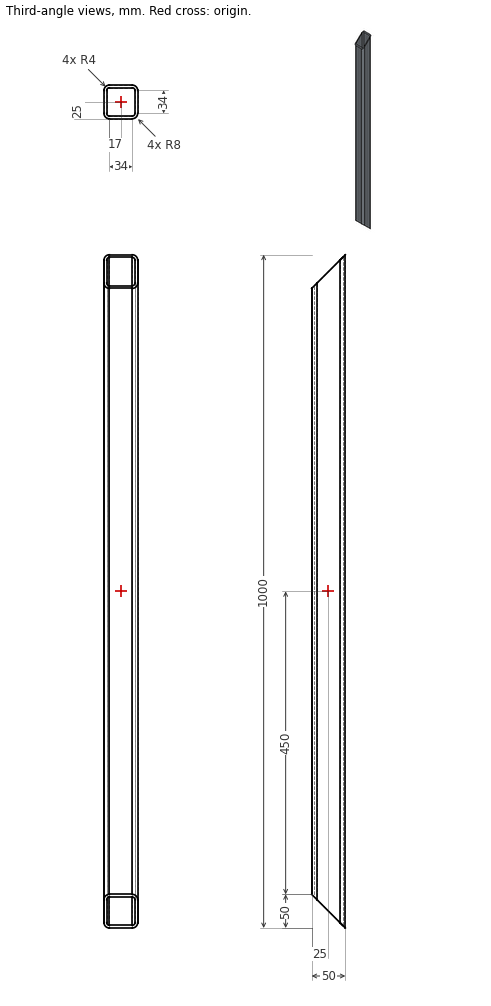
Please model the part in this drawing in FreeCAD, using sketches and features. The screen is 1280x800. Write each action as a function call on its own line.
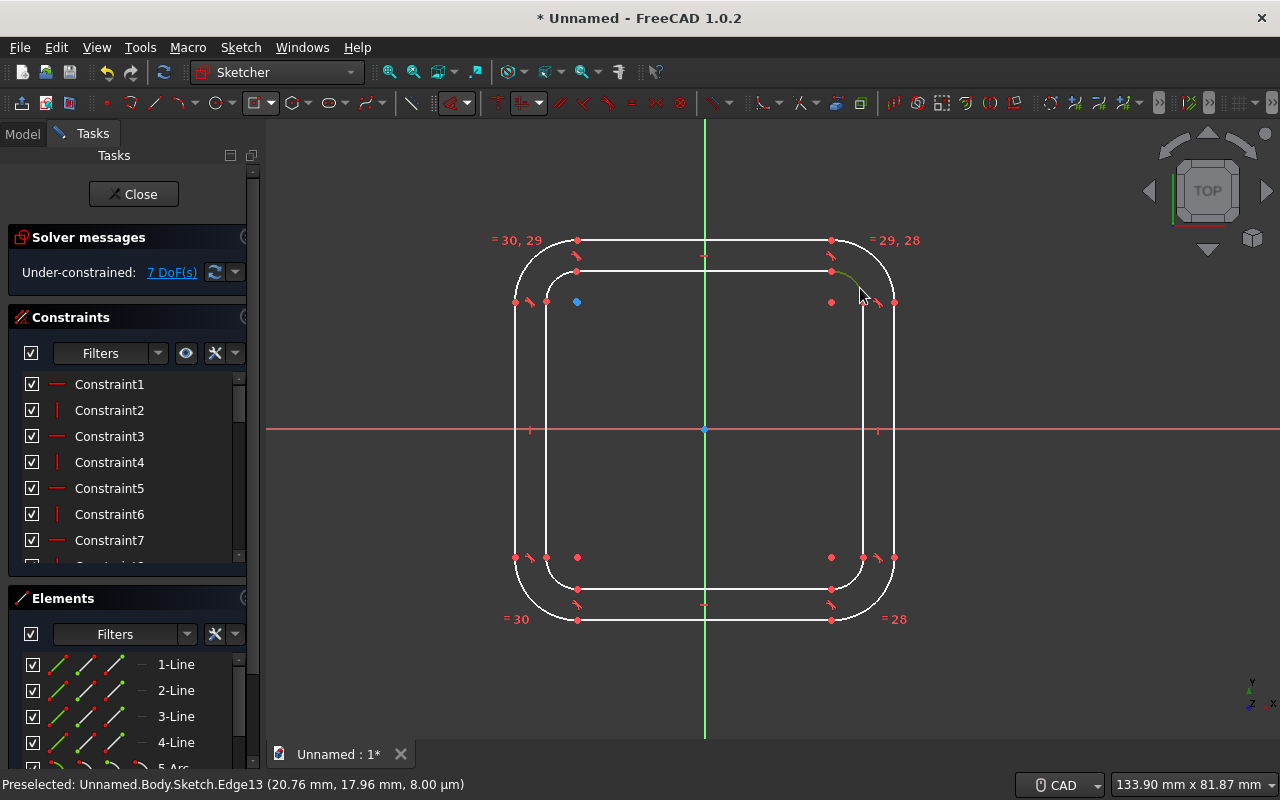
click(563, 275)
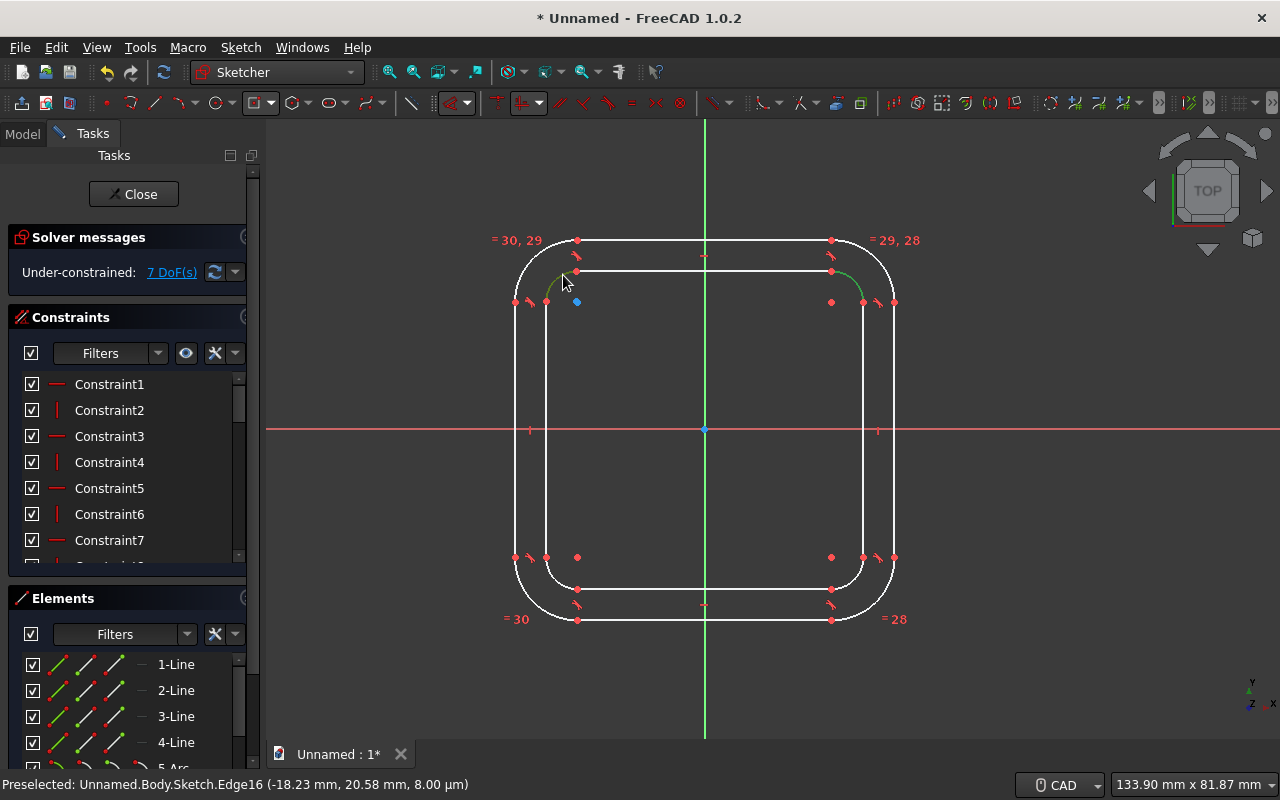
key(e)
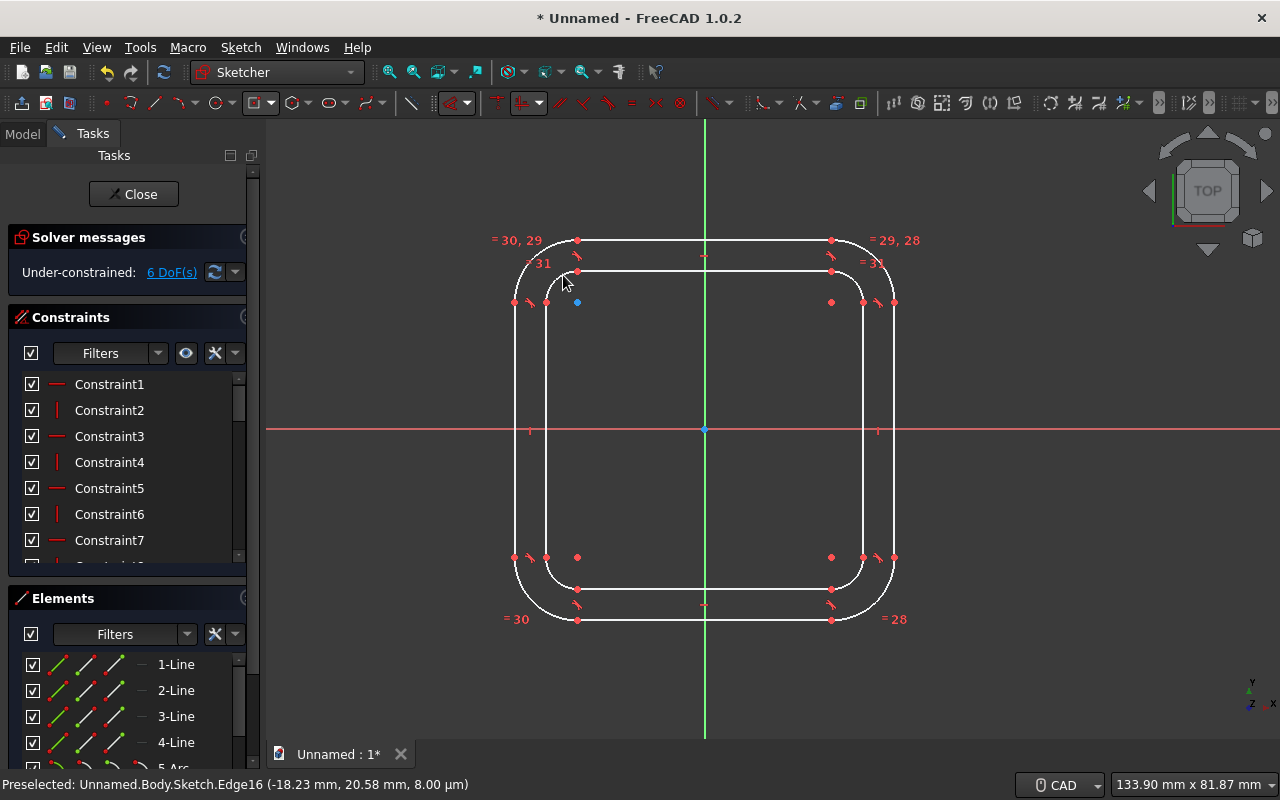
key(d)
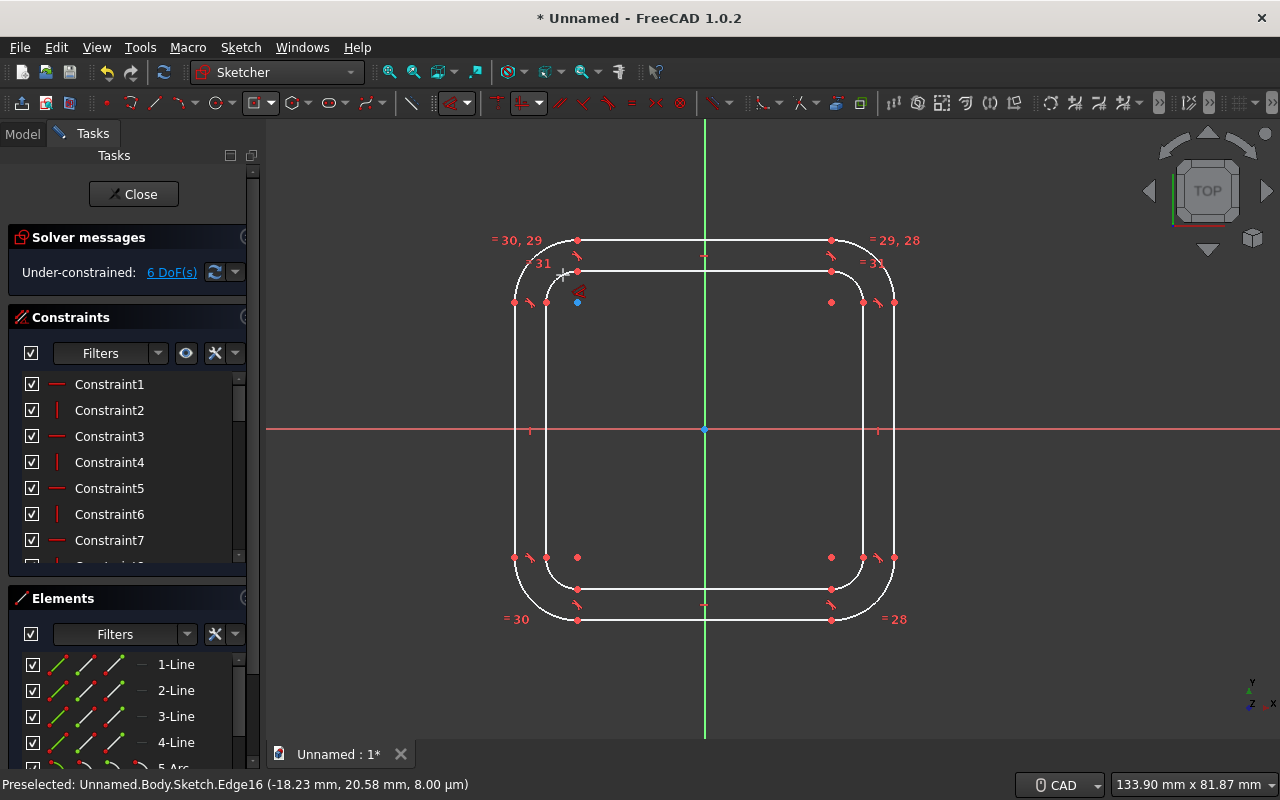
click(860, 614)
click(874, 643)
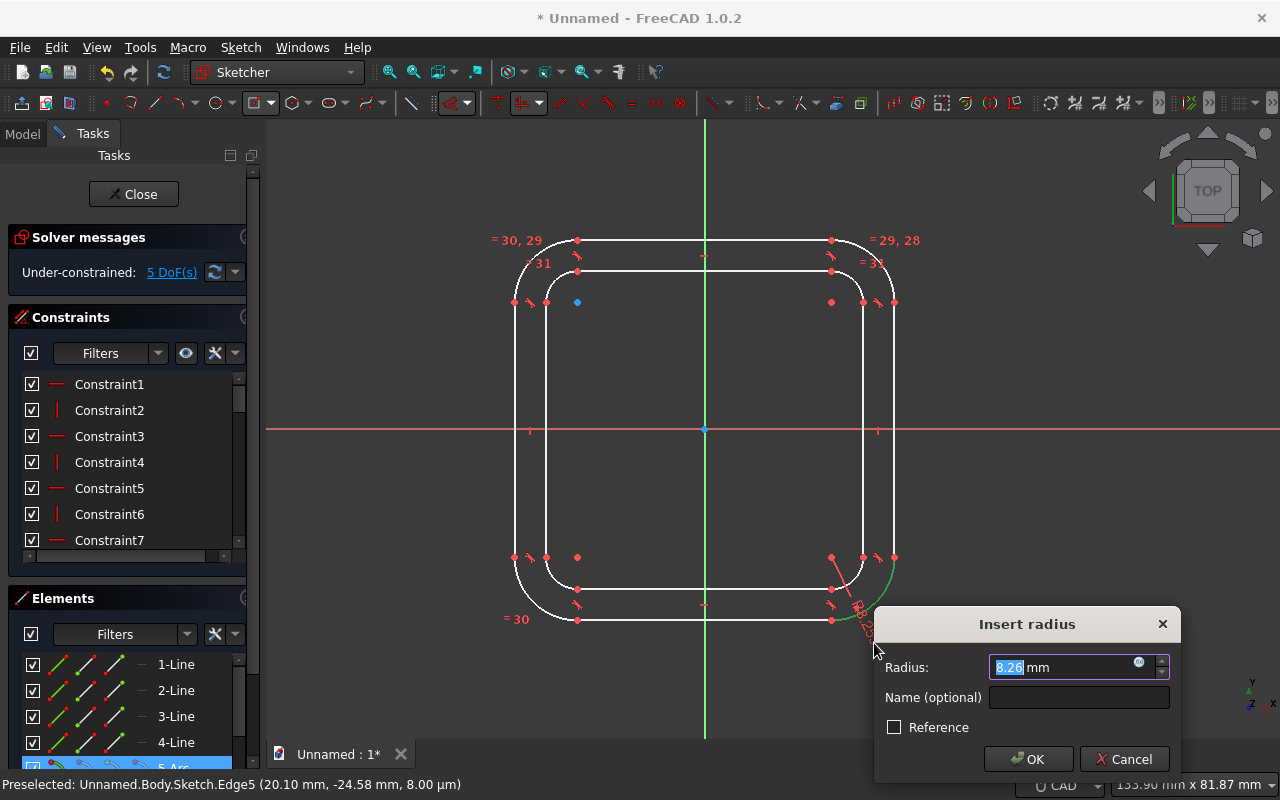
text(8)
key(Return)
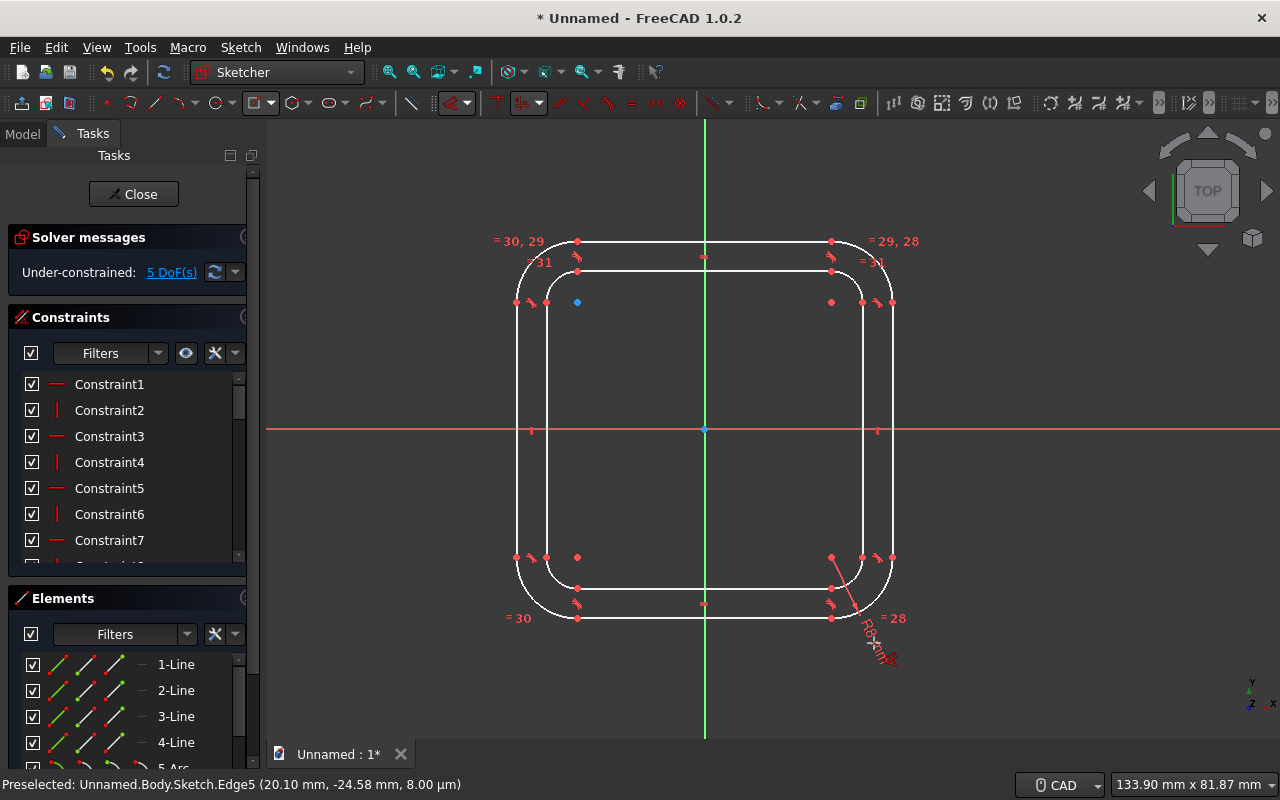
scroll(859, 288, up, 2)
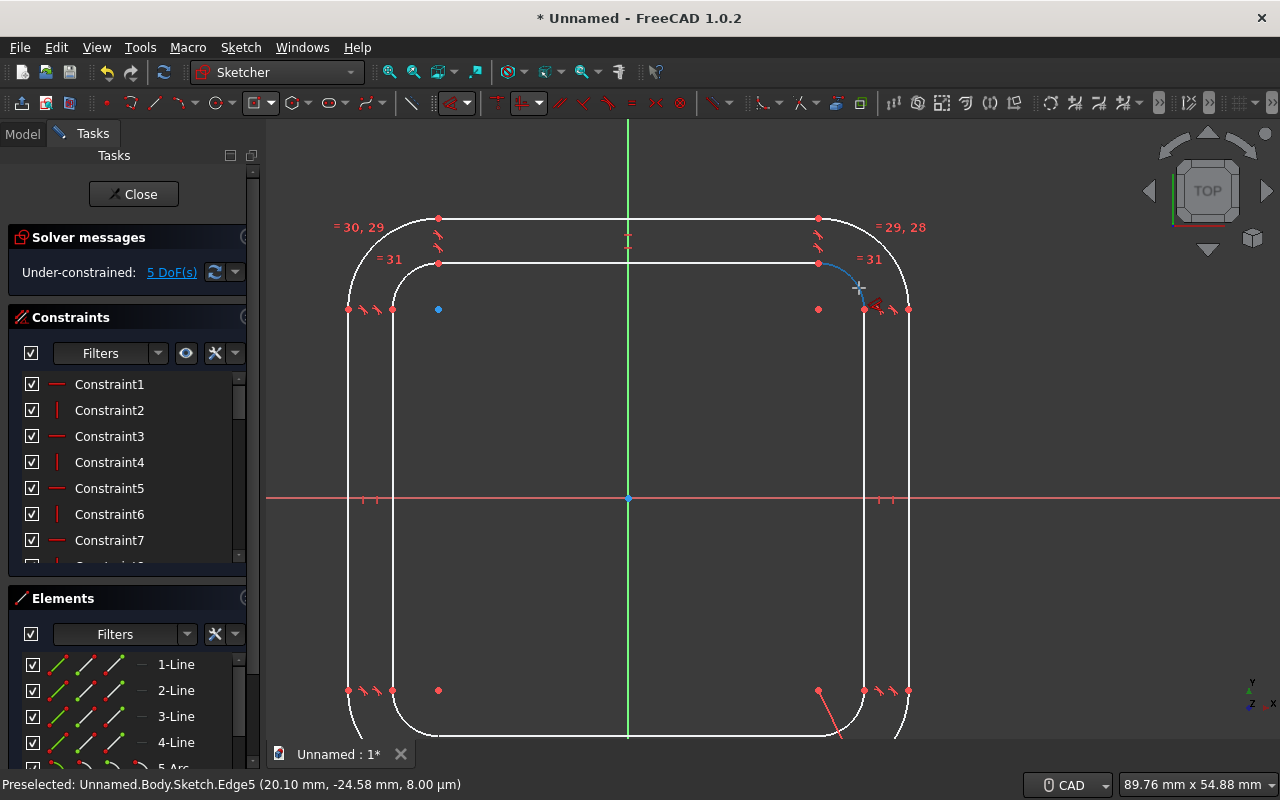
click(859, 288)
click(886, 348)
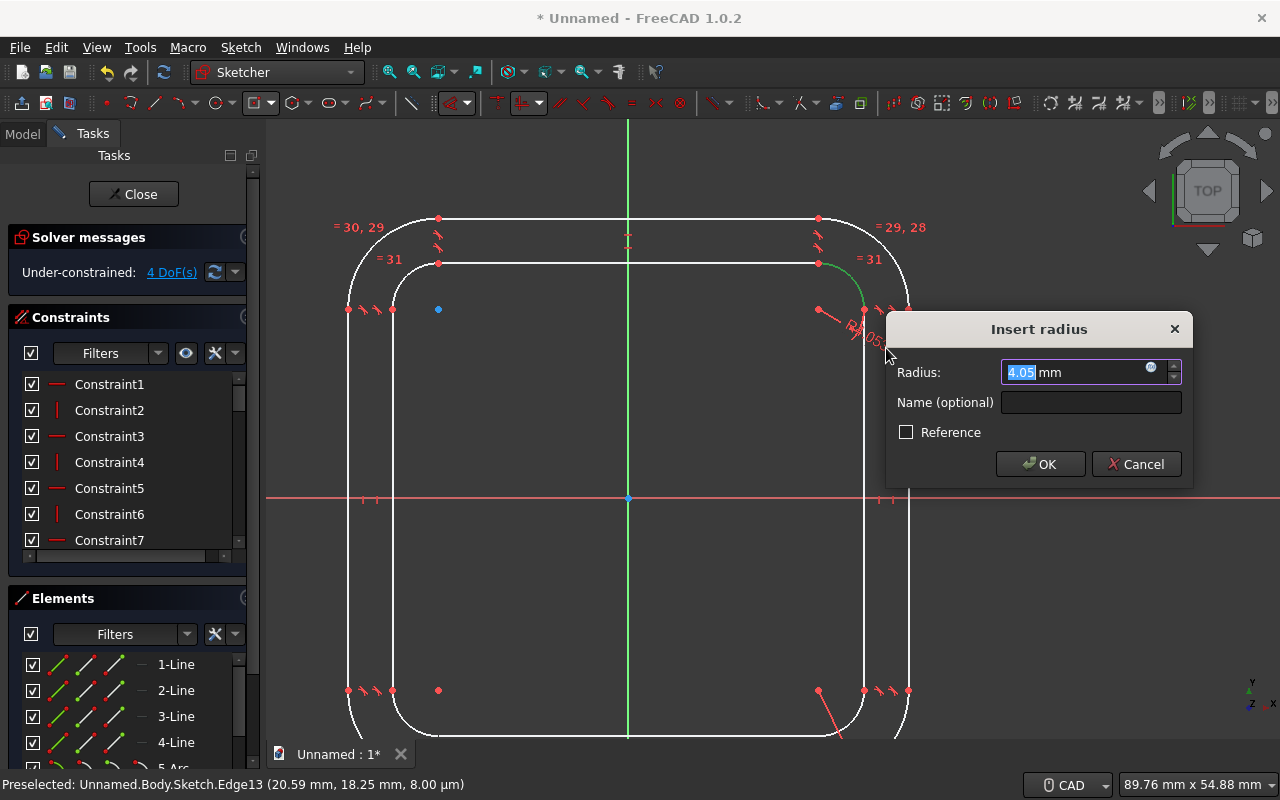
text(4)
key(Return)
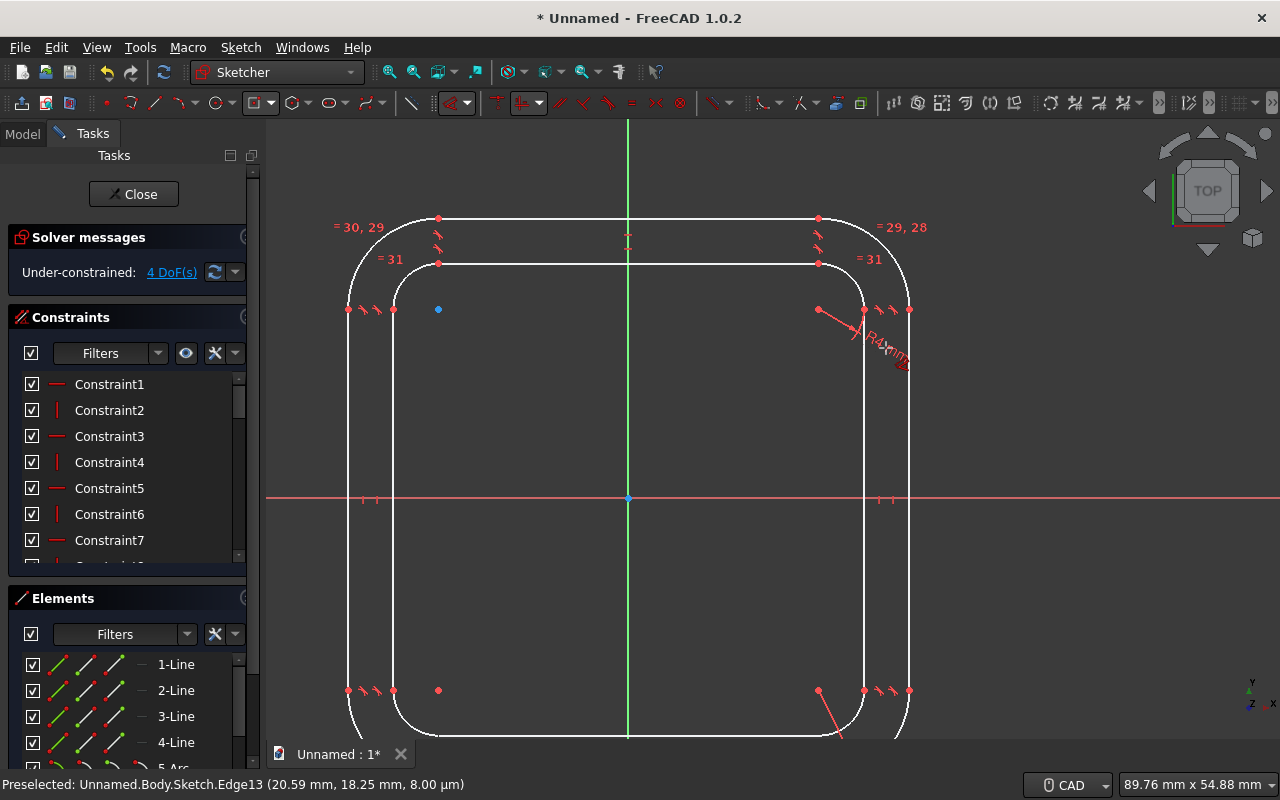
scroll(859, 288, down, 2)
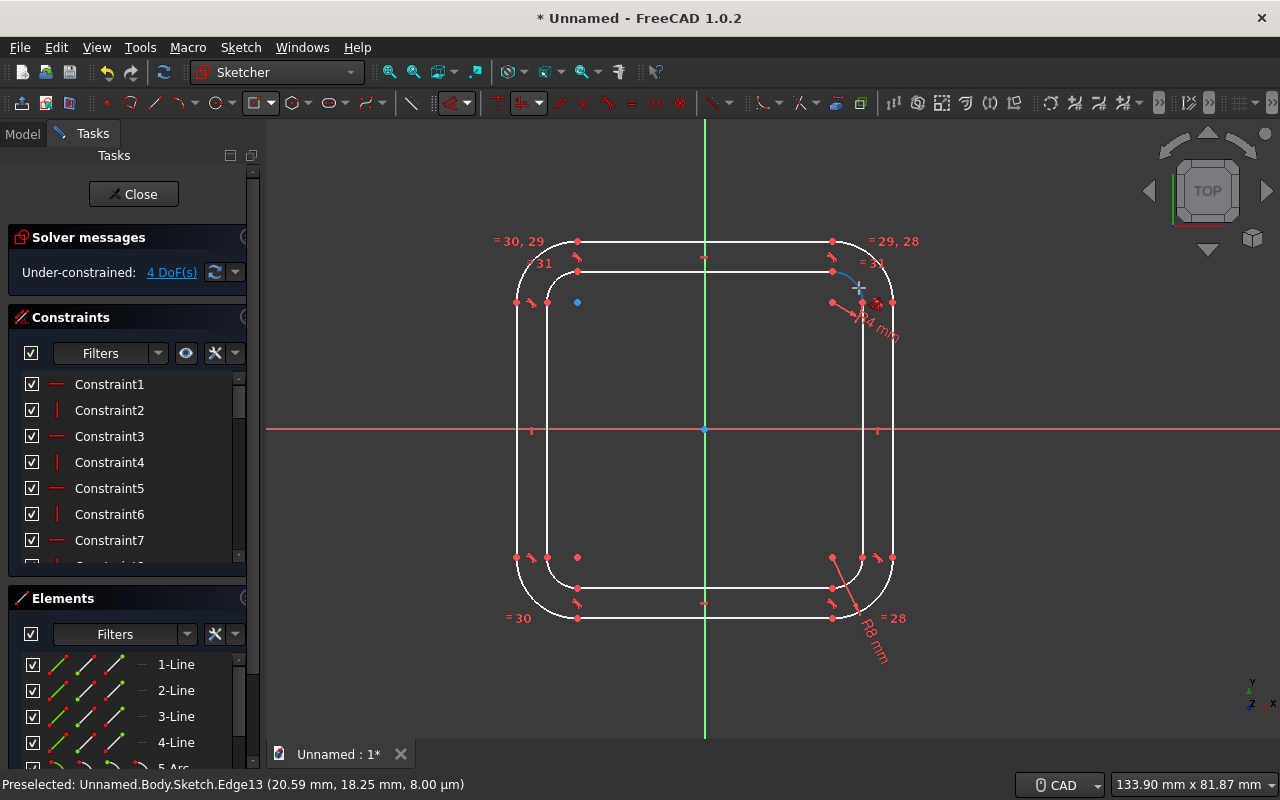
click(654, 618)
click(646, 652)